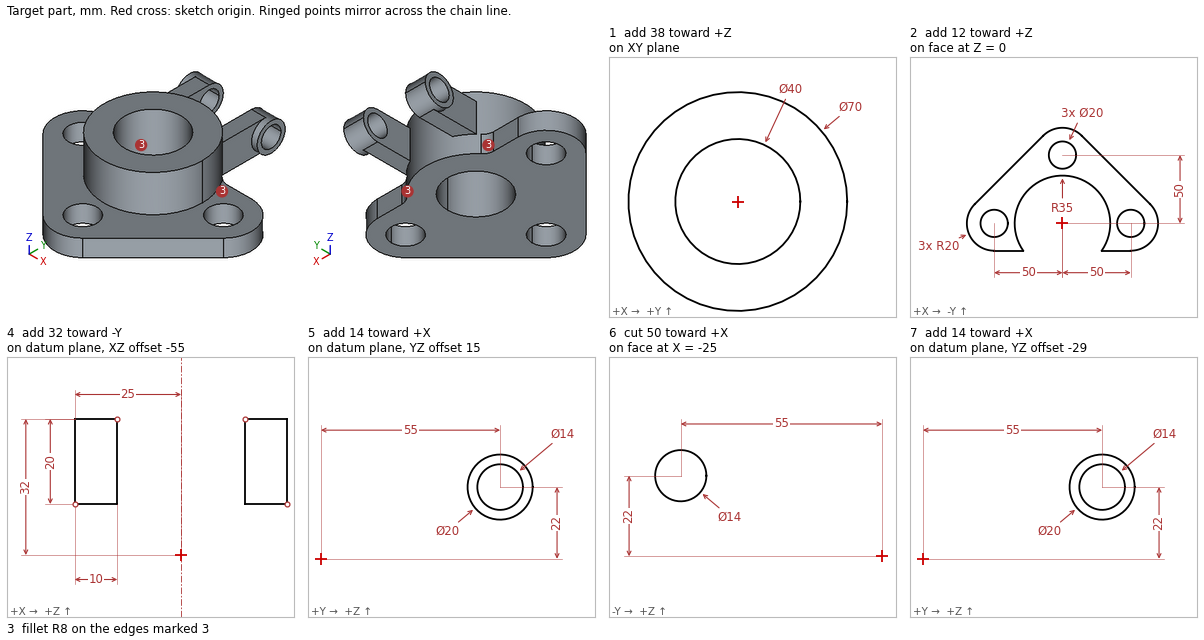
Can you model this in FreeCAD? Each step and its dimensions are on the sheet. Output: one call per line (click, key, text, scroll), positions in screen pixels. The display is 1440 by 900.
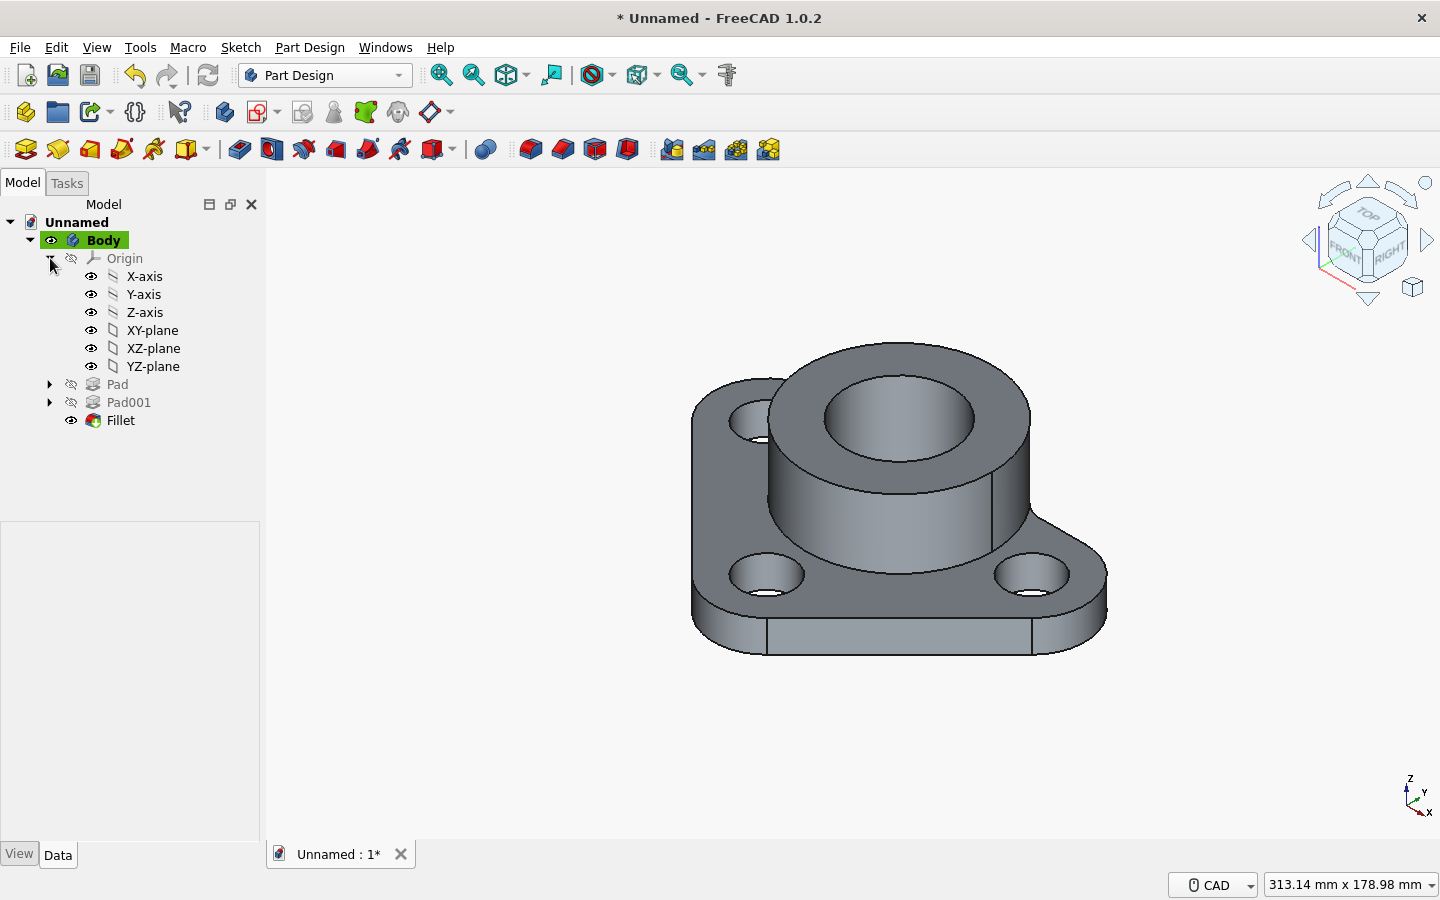
click(136, 348)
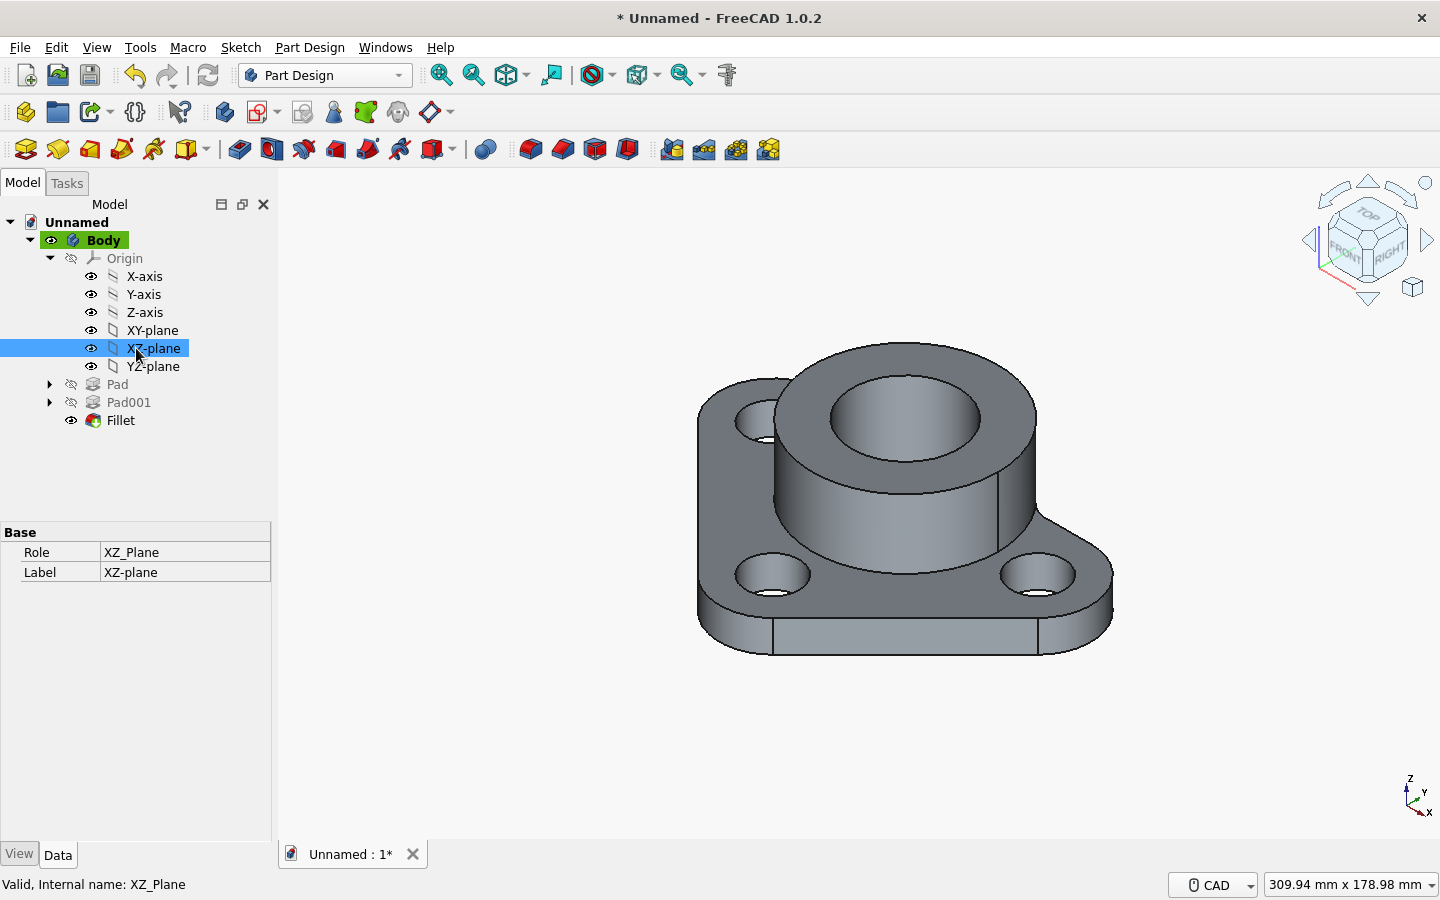
click(430, 112)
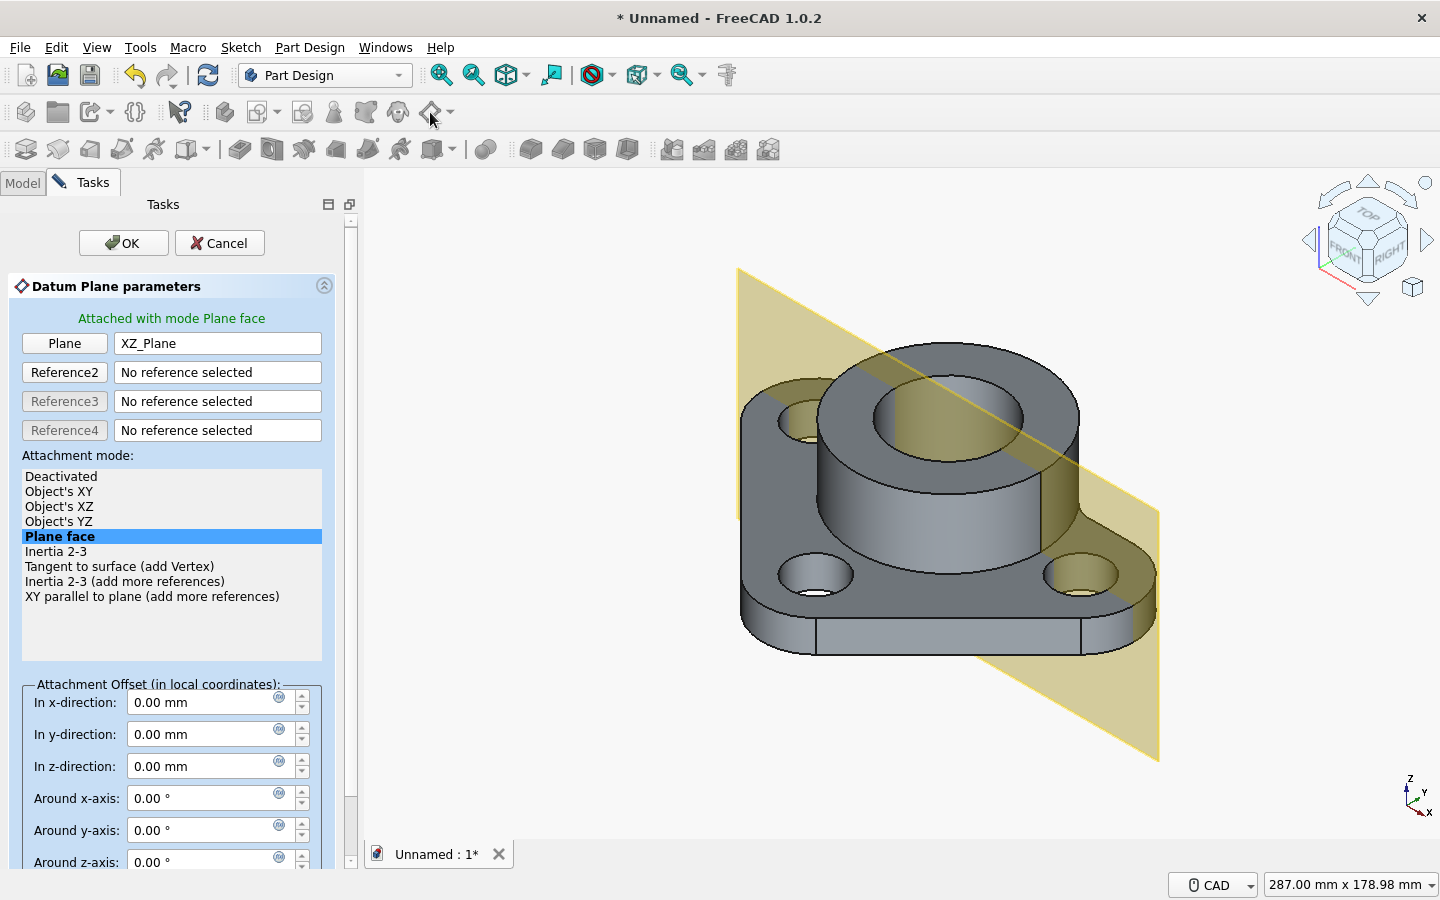
triple_click(210, 766)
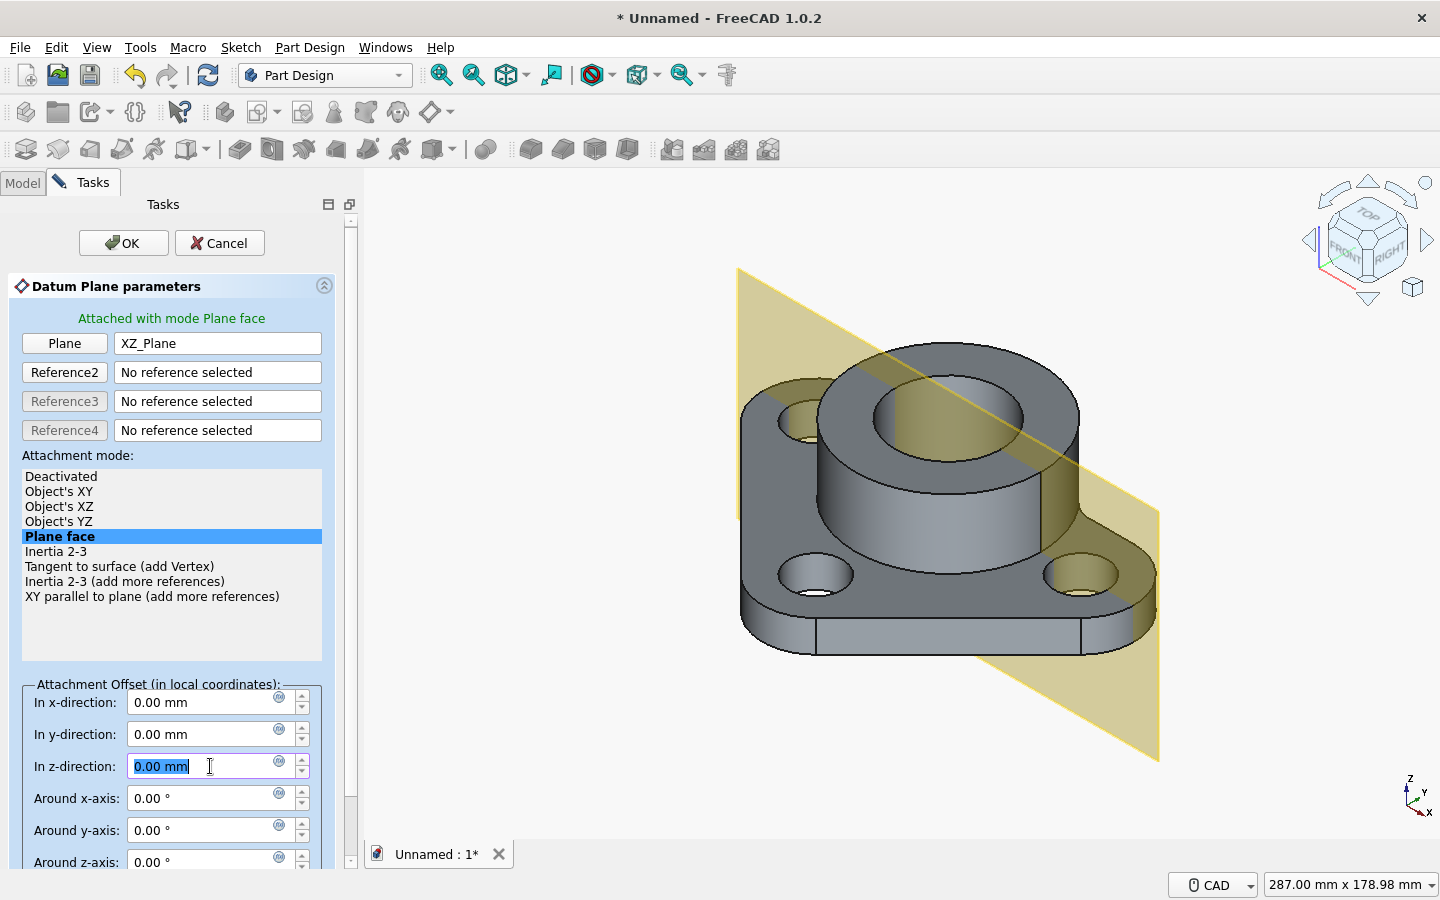
text(-55)
key(Tab)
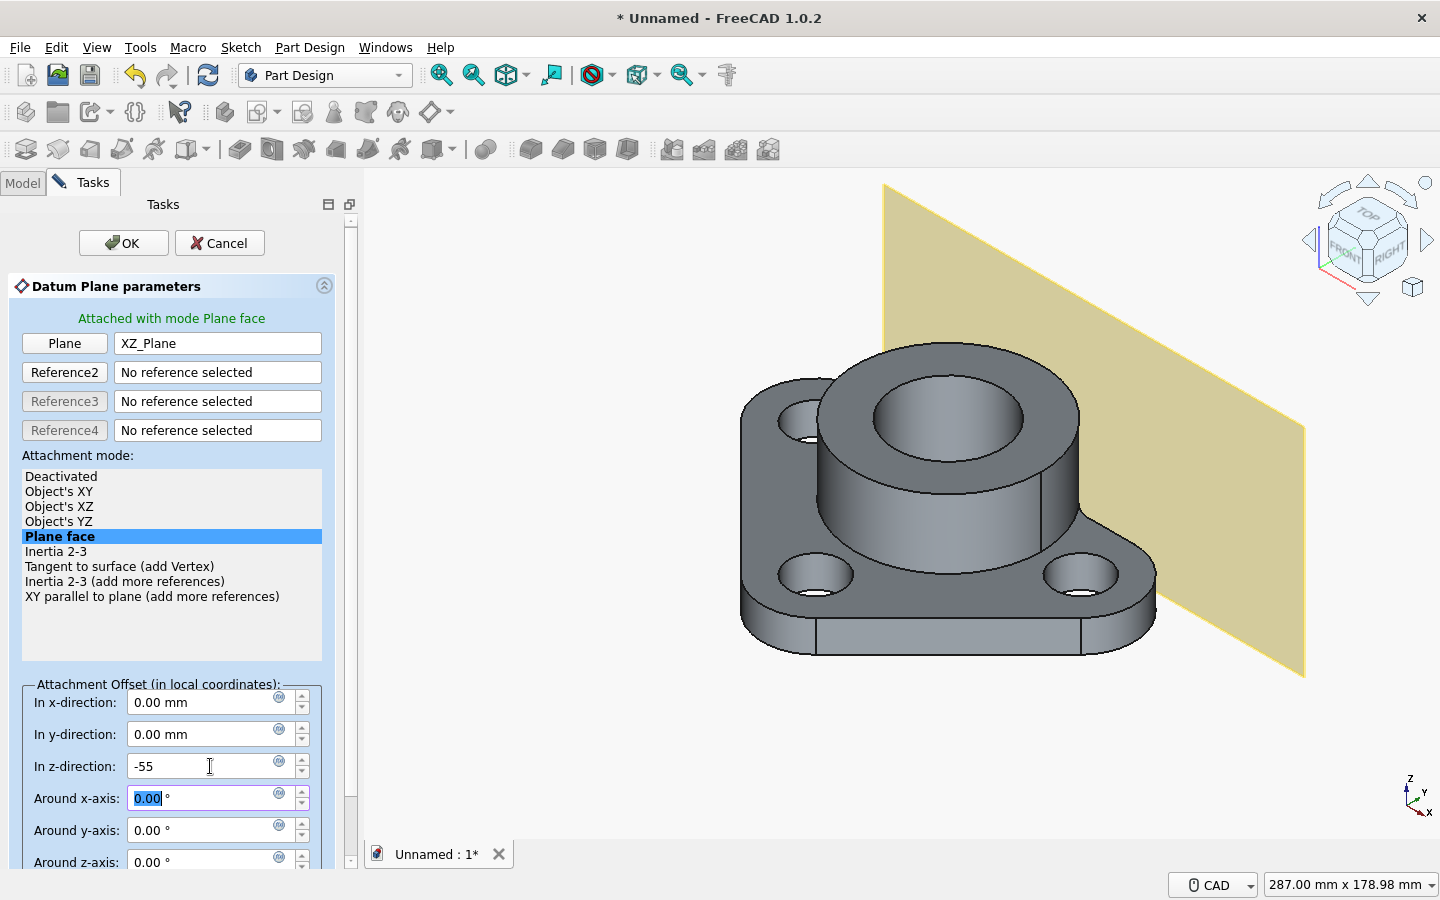
click(124, 243)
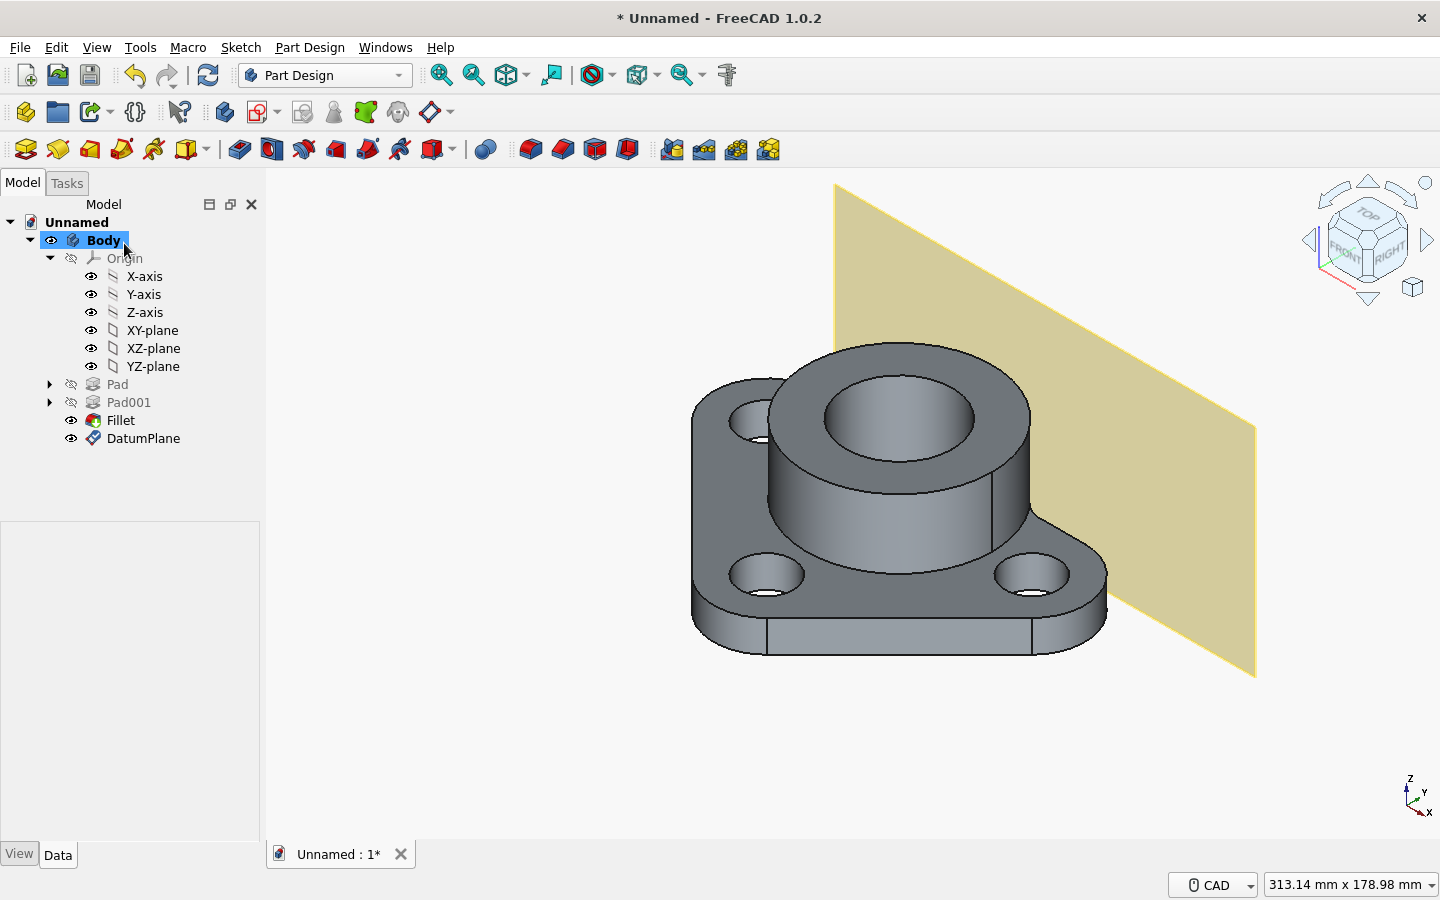
click(116, 438)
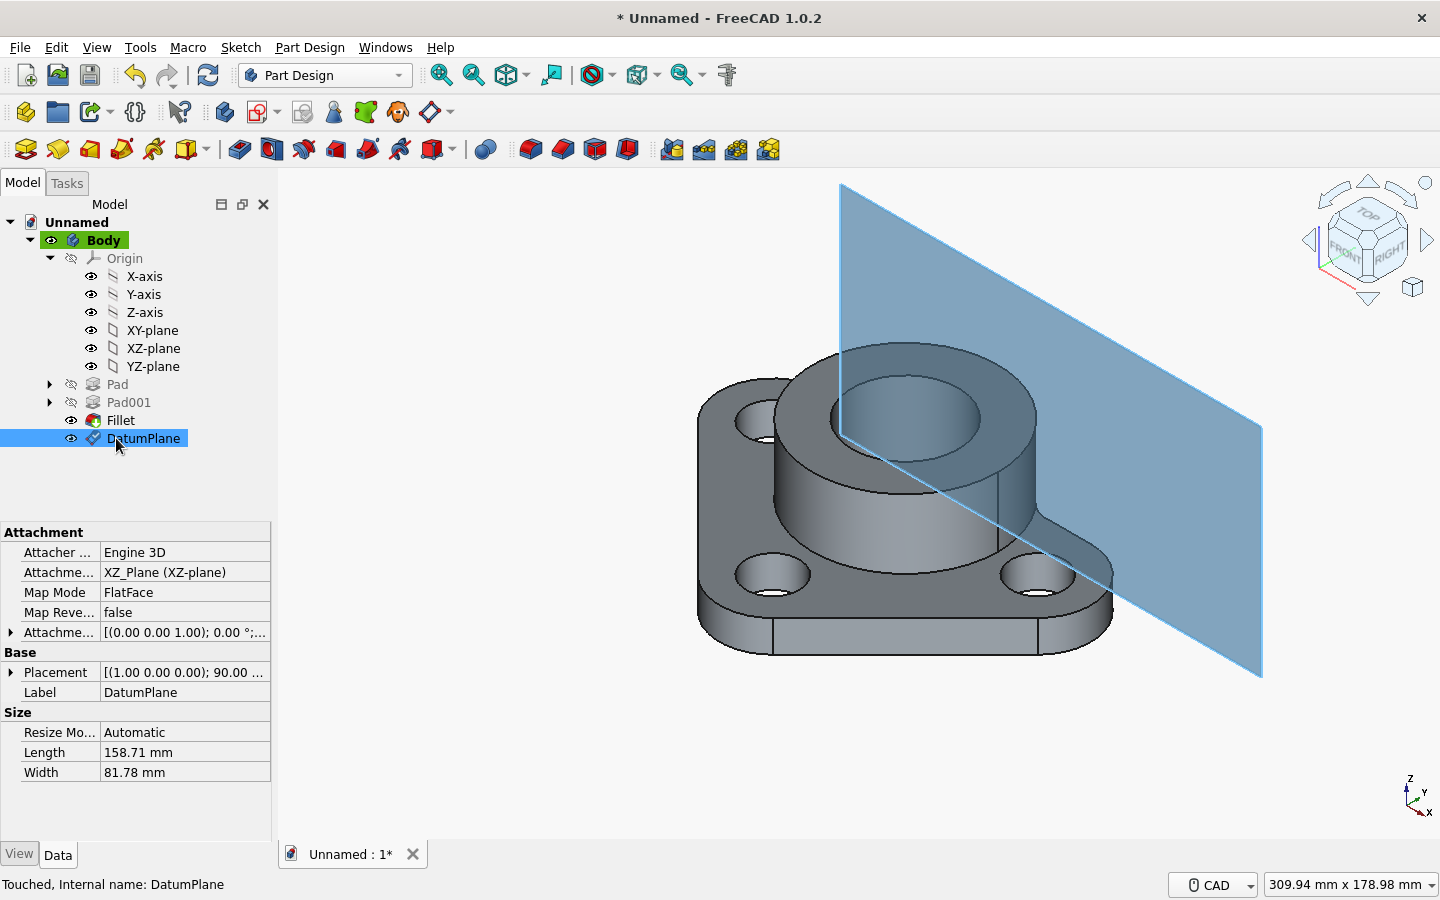
click(258, 112)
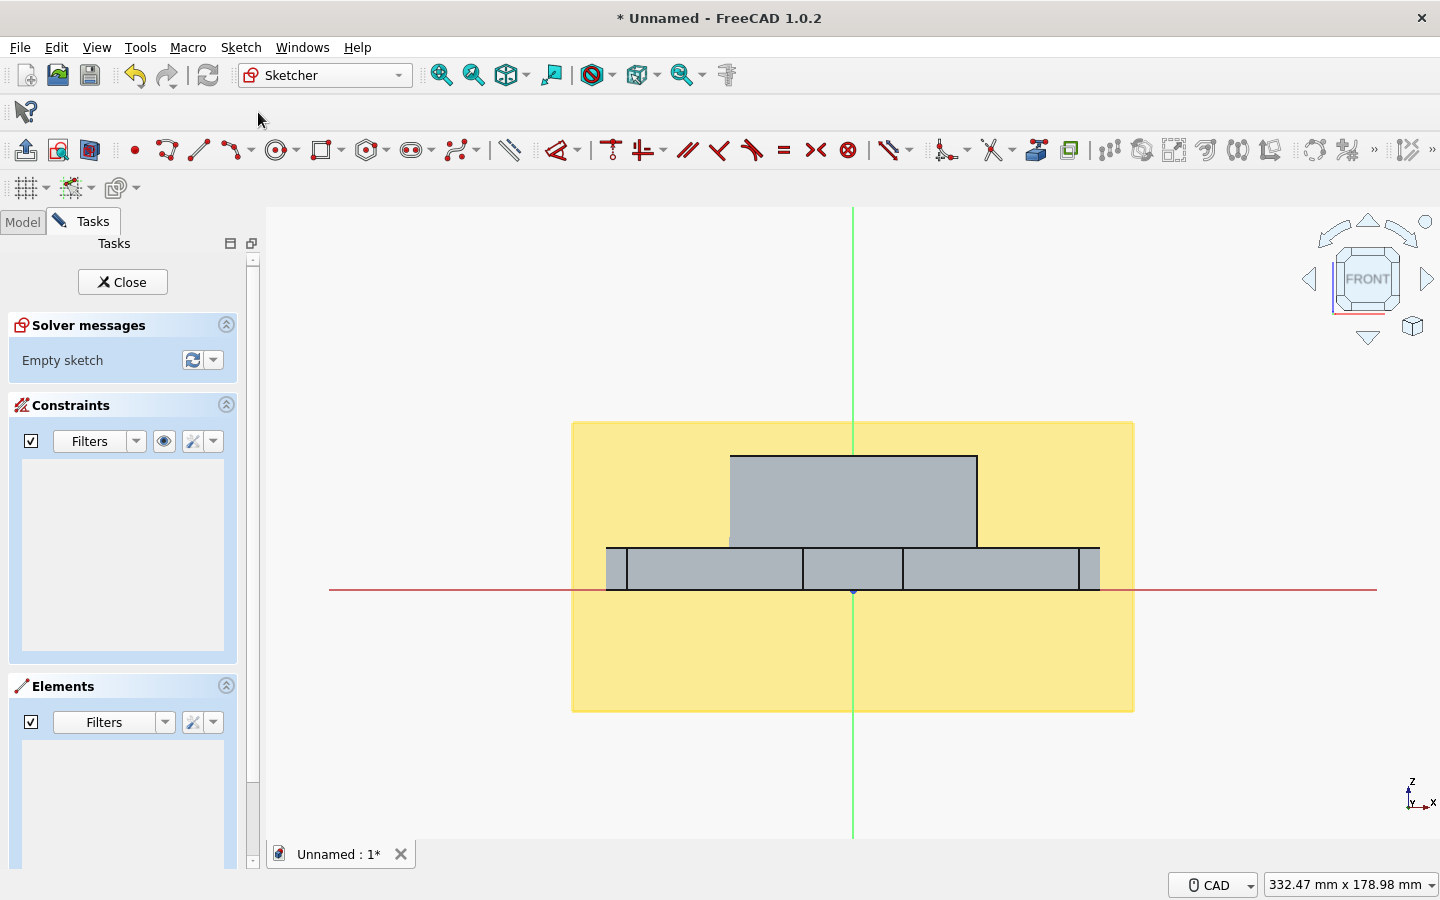
key(q)
key(s)